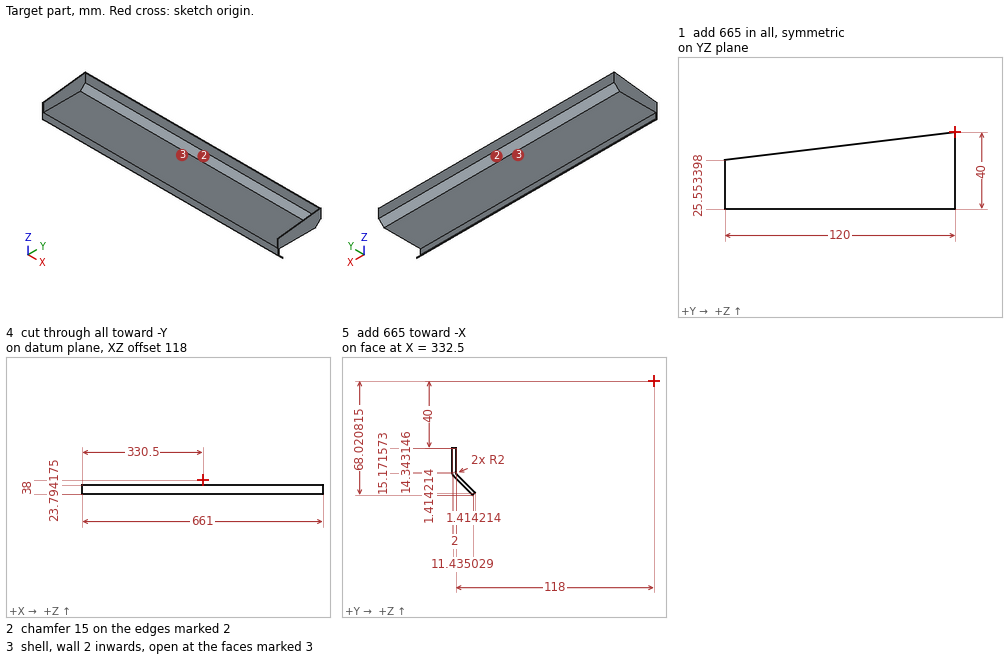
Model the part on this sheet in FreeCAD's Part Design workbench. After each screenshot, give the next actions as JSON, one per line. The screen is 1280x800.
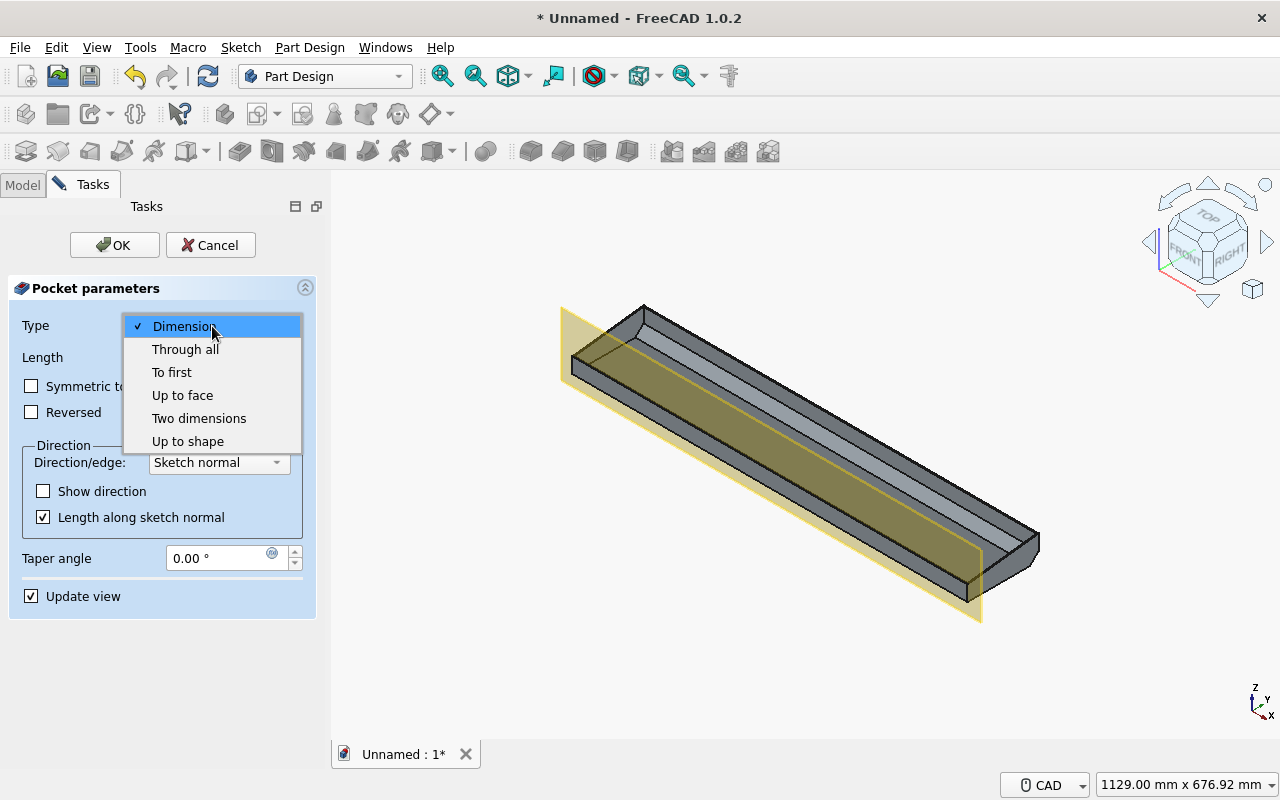
{"action": "left_click", "coordinate": [212, 350]}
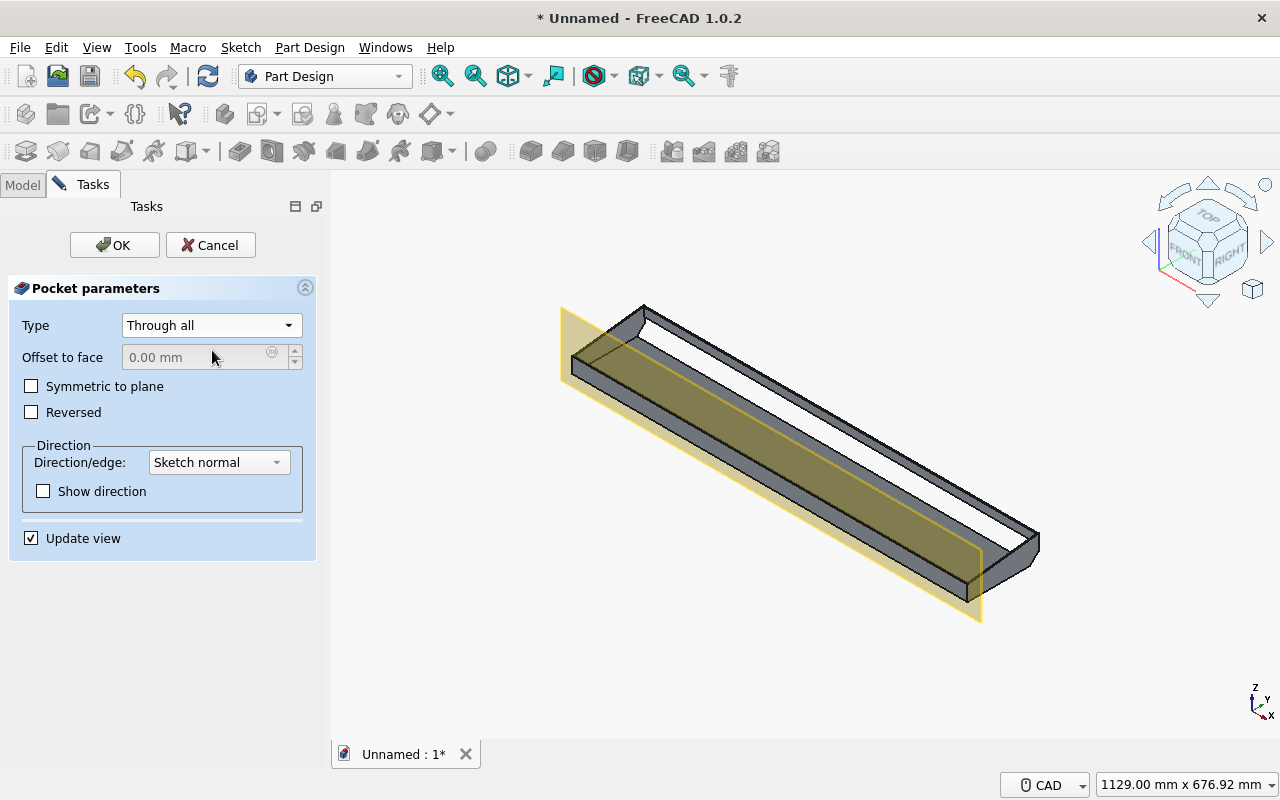
{"action": "left_click", "coordinate": [30, 412]}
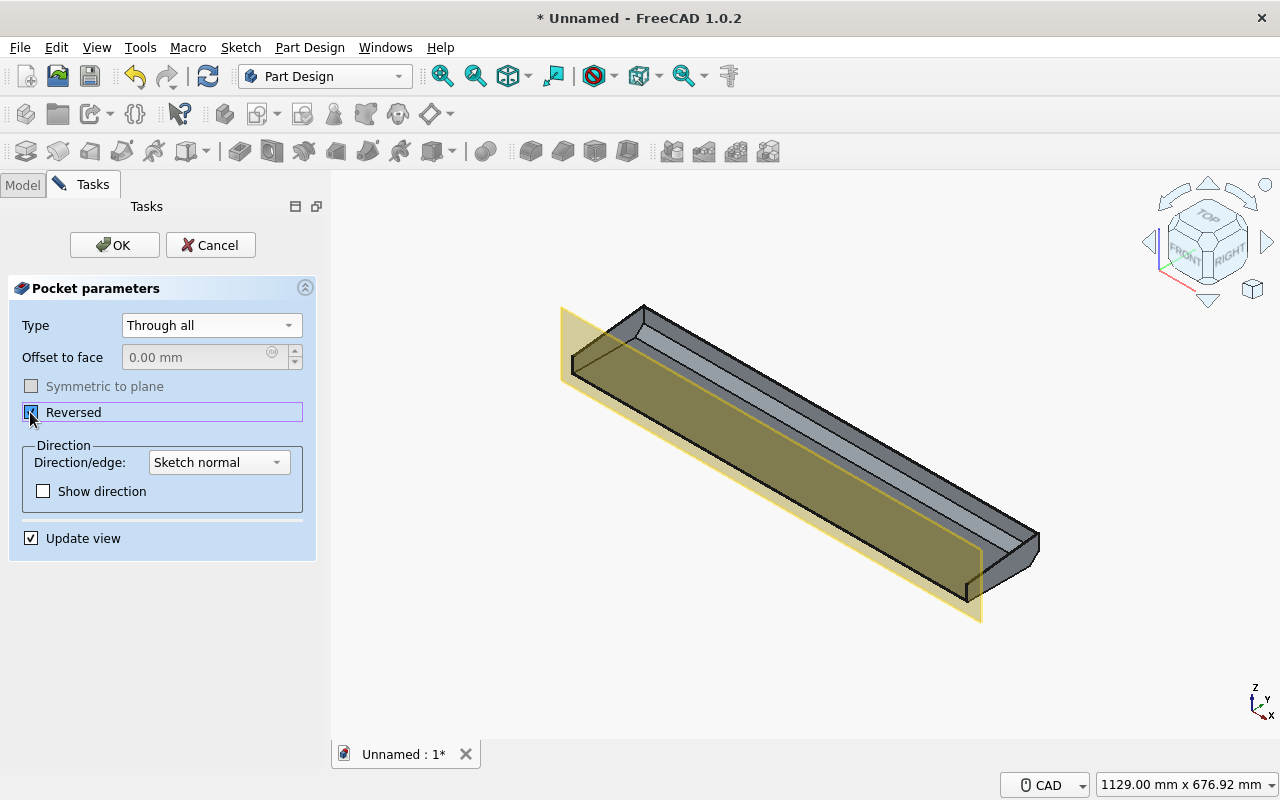
{"action": "left_click", "coordinate": [115, 245]}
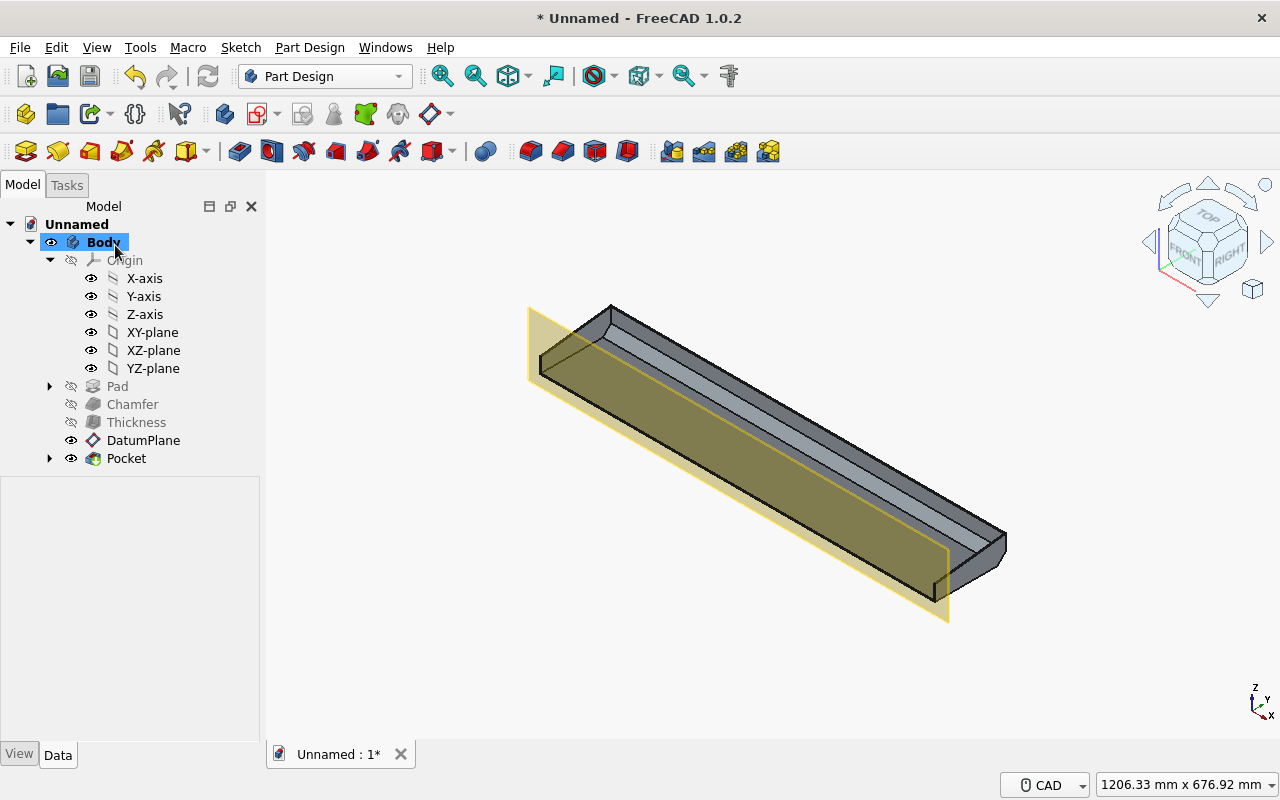
{"action": "left_click", "coordinate": [116, 440]}
{"action": "key", "text": "space"}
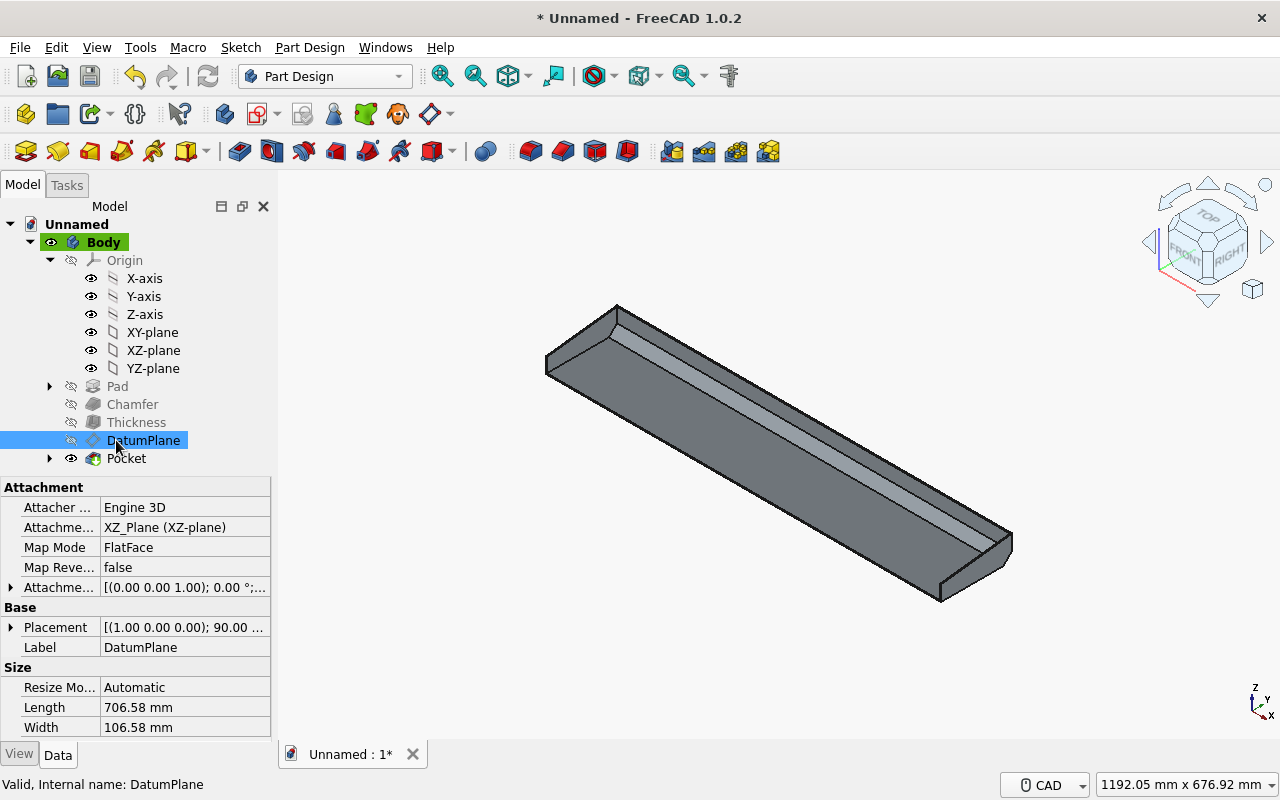
{"action": "left_click", "coordinate": [997, 555]}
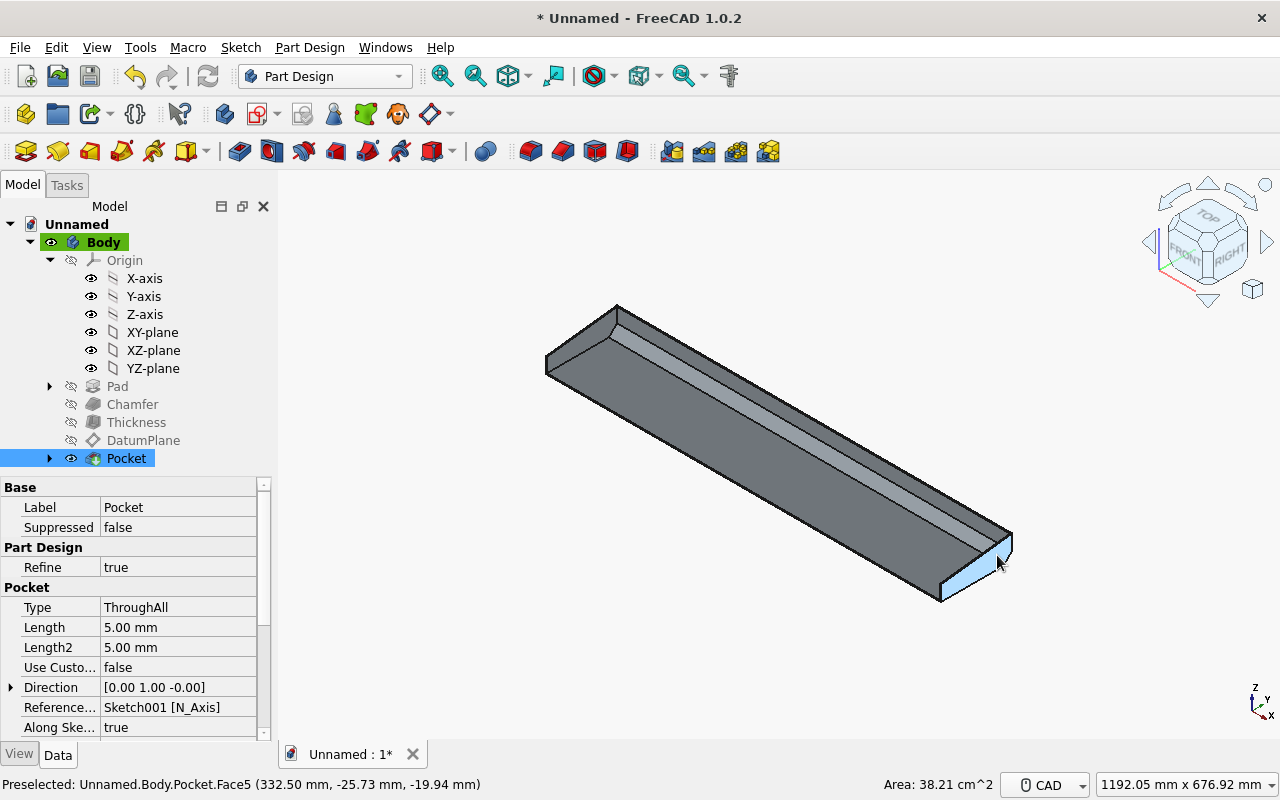
{"action": "left_click", "coordinate": [258, 114]}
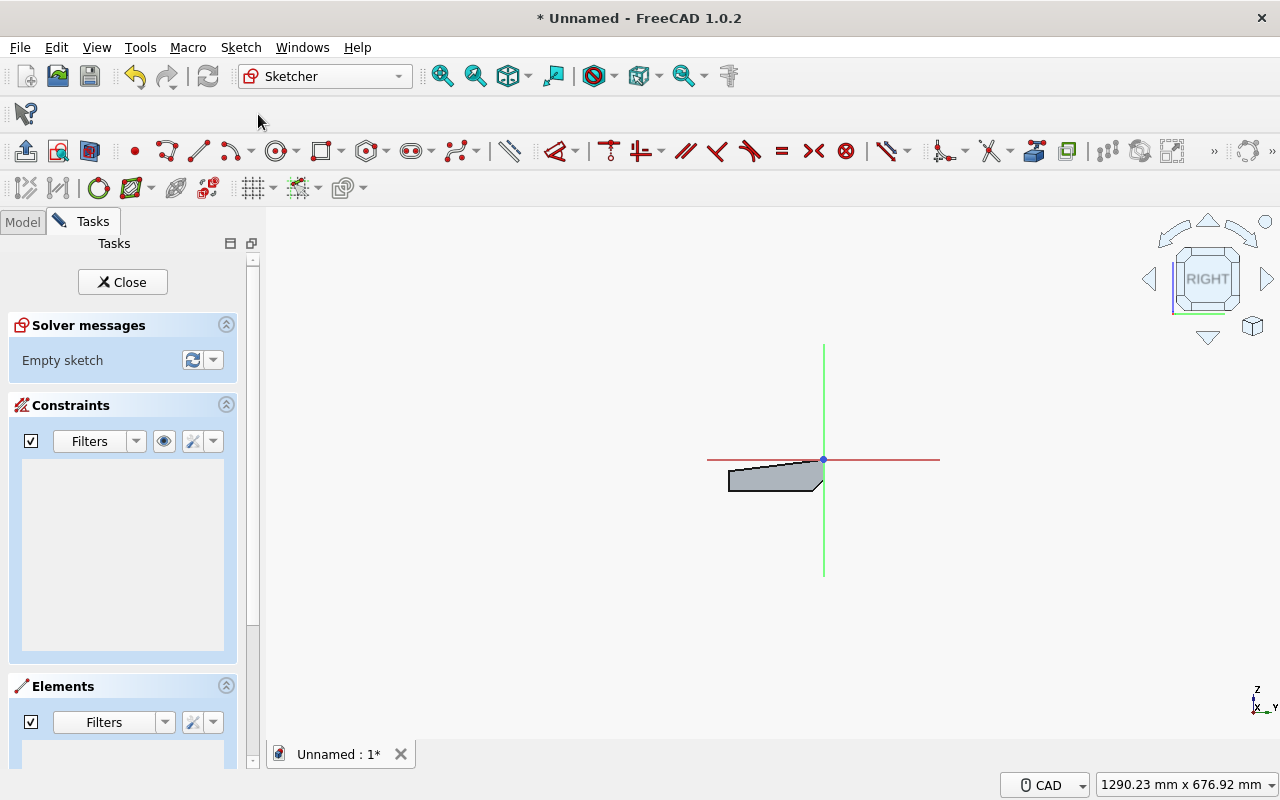
{"action": "scroll", "coordinate": [737, 504], "scroll_direction": "up", "scroll_amount": 14}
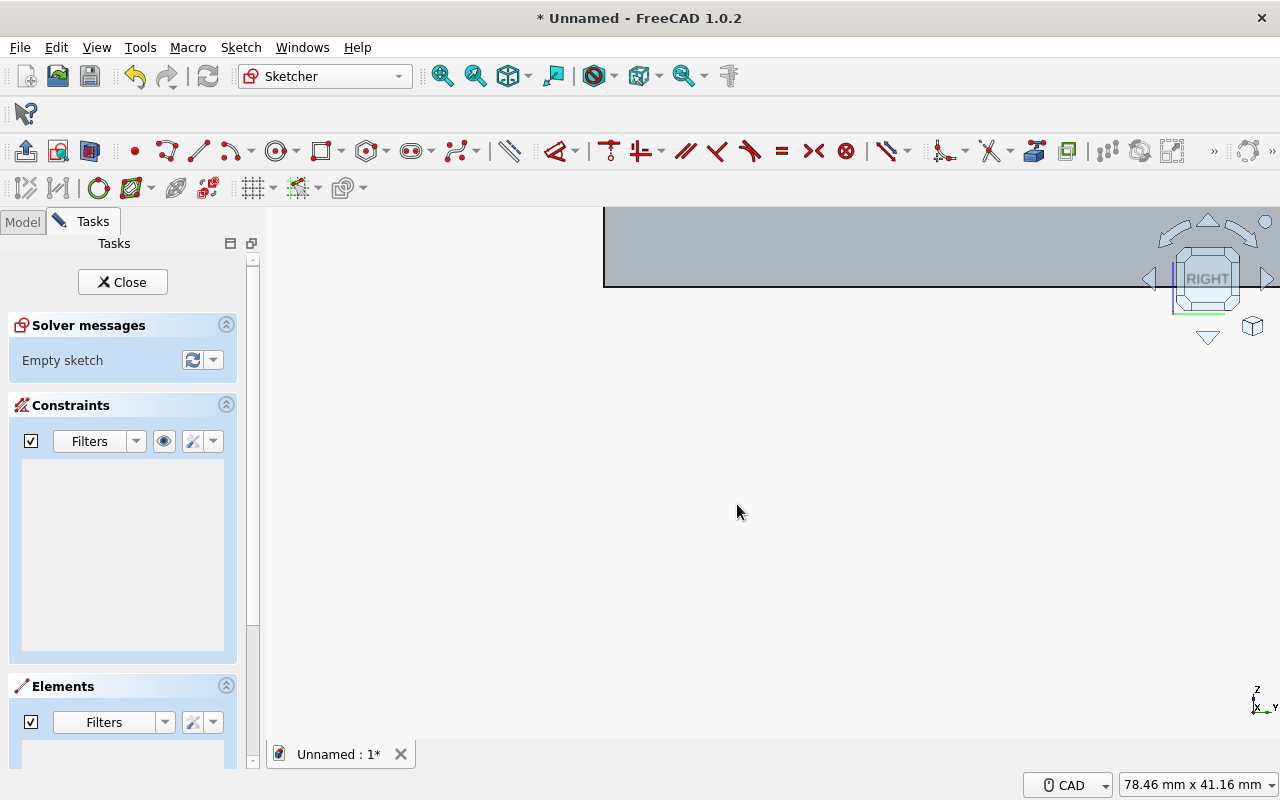
{"action": "key", "text": "g m"}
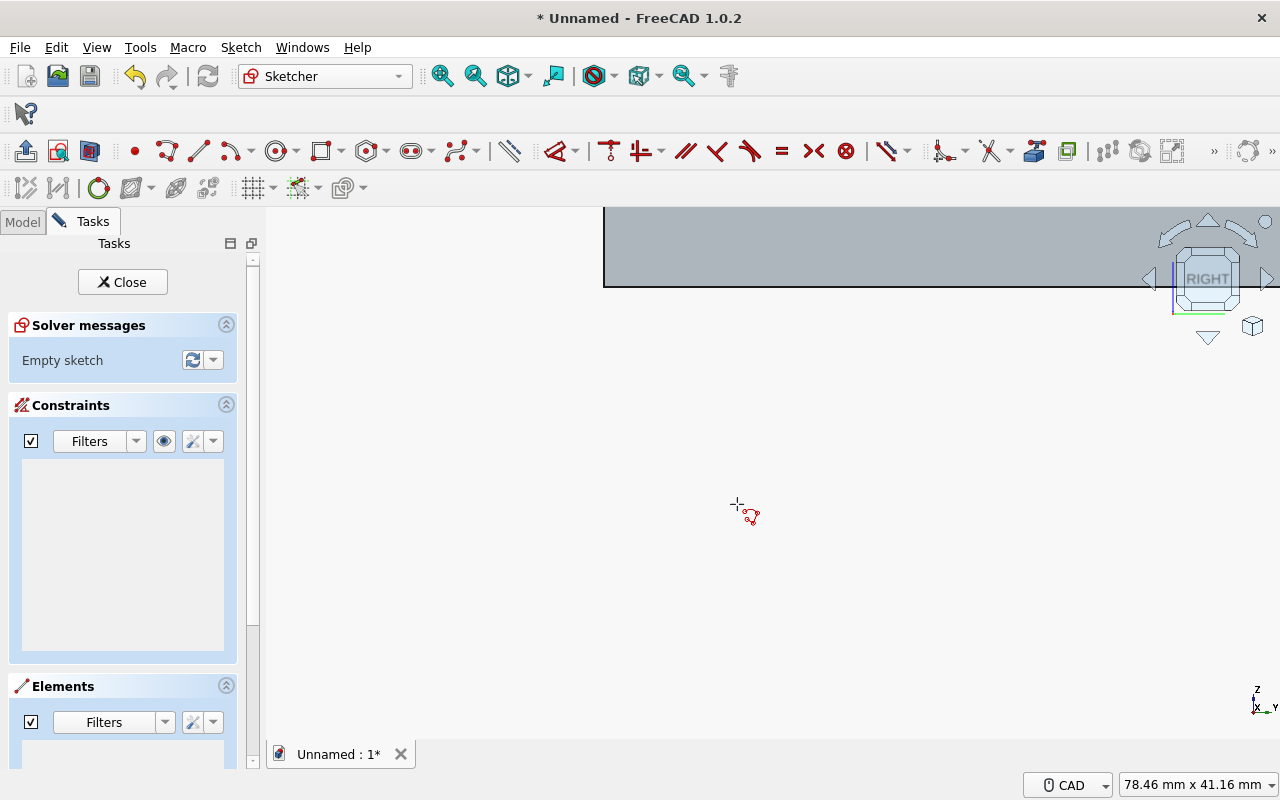
{"action": "left_click", "coordinate": [612, 501]}
{"action": "left_click", "coordinate": [759, 649]}
{"action": "left_click", "coordinate": [778, 630]}
{"action": "left_click", "coordinate": [637, 490]}
{"action": "right_click", "coordinate": [637, 490]}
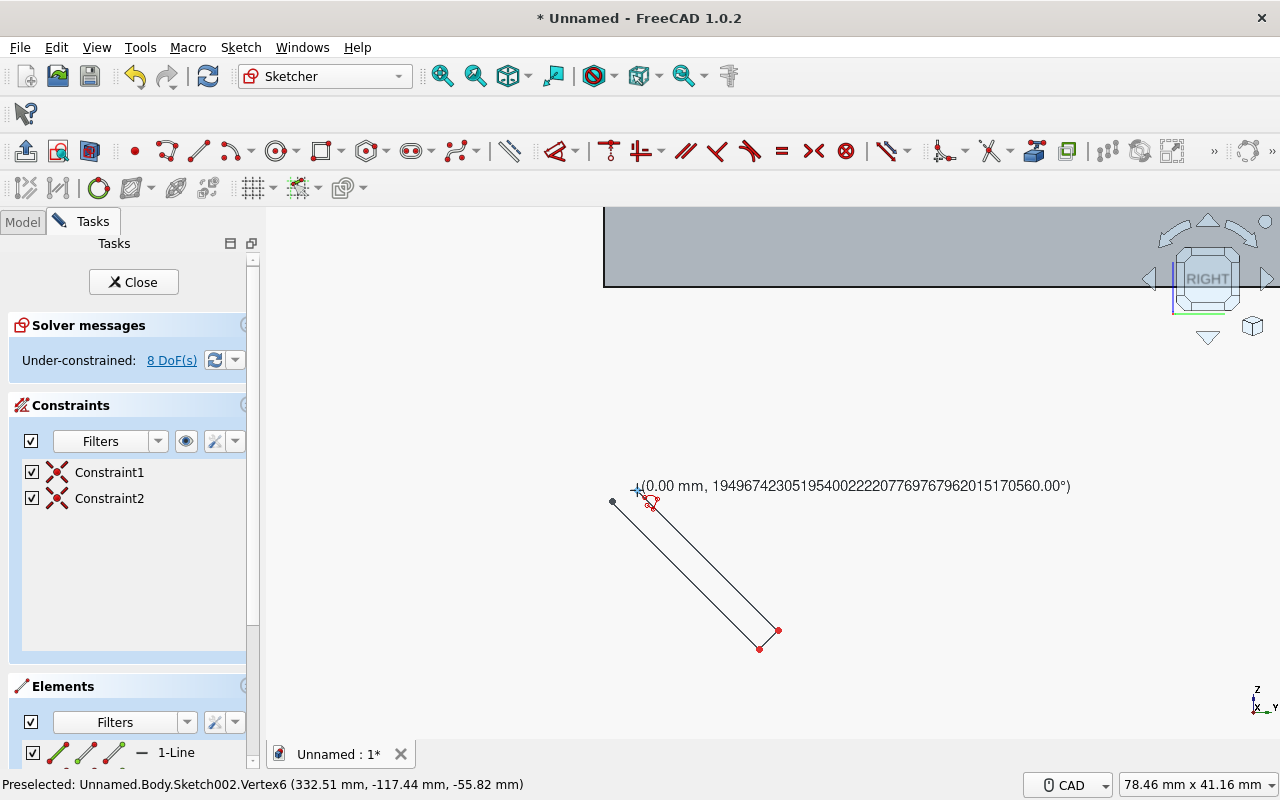
{"action": "left_click", "coordinate": [630, 472]}
{"action": "left_click", "coordinate": [630, 287]}
{"action": "left_click", "coordinate": [604, 287]}
{"action": "left_click", "coordinate": [604, 483]}
{"action": "right_click", "coordinate": [604, 483]}